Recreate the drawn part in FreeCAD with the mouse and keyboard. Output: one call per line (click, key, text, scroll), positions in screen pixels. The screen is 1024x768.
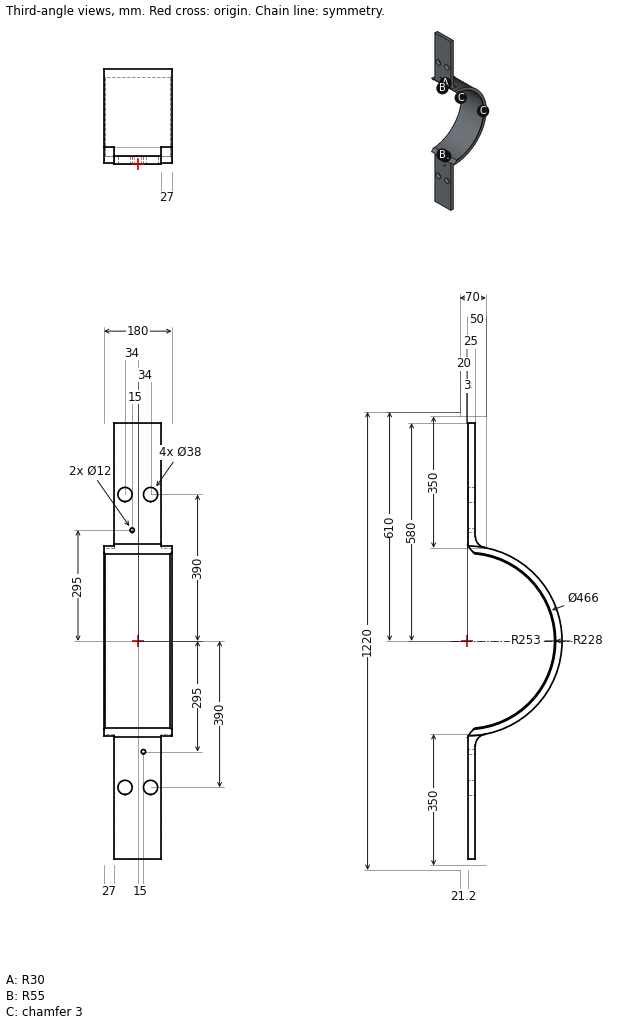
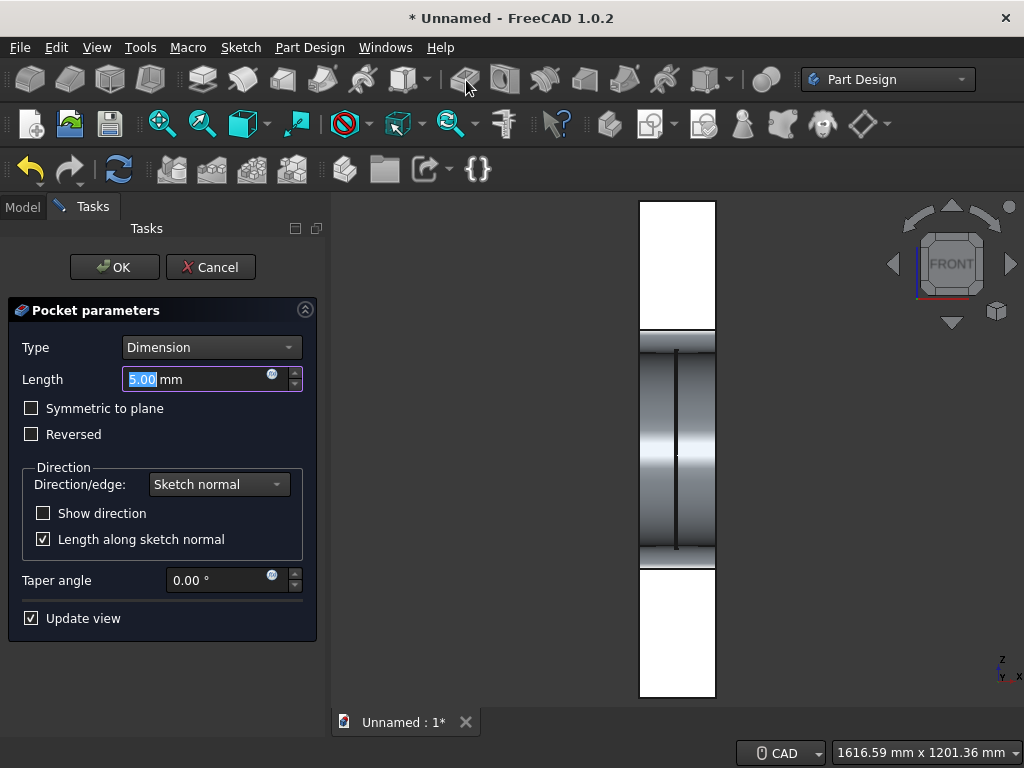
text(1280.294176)
key(Tab)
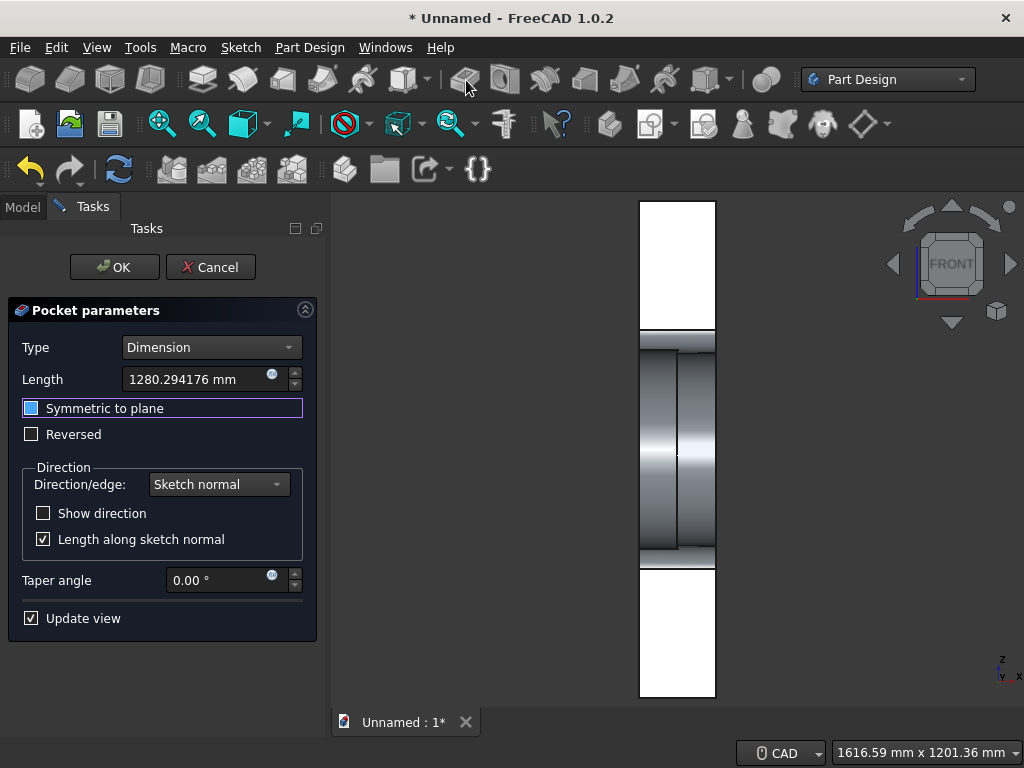
click(30, 408)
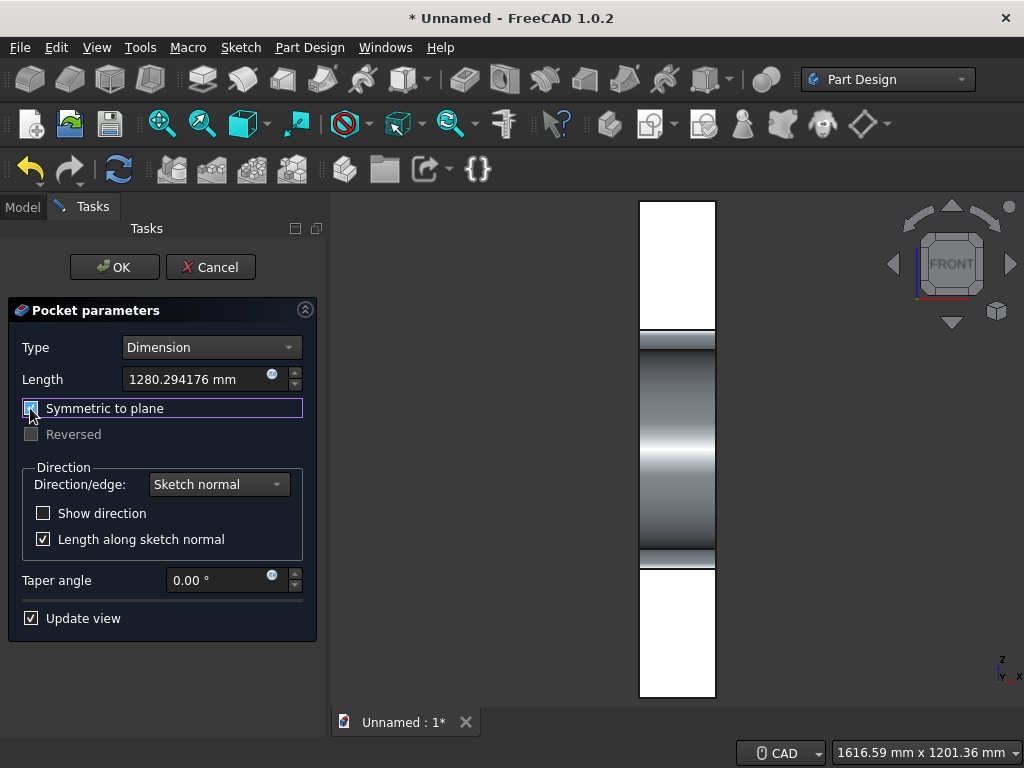
click(115, 267)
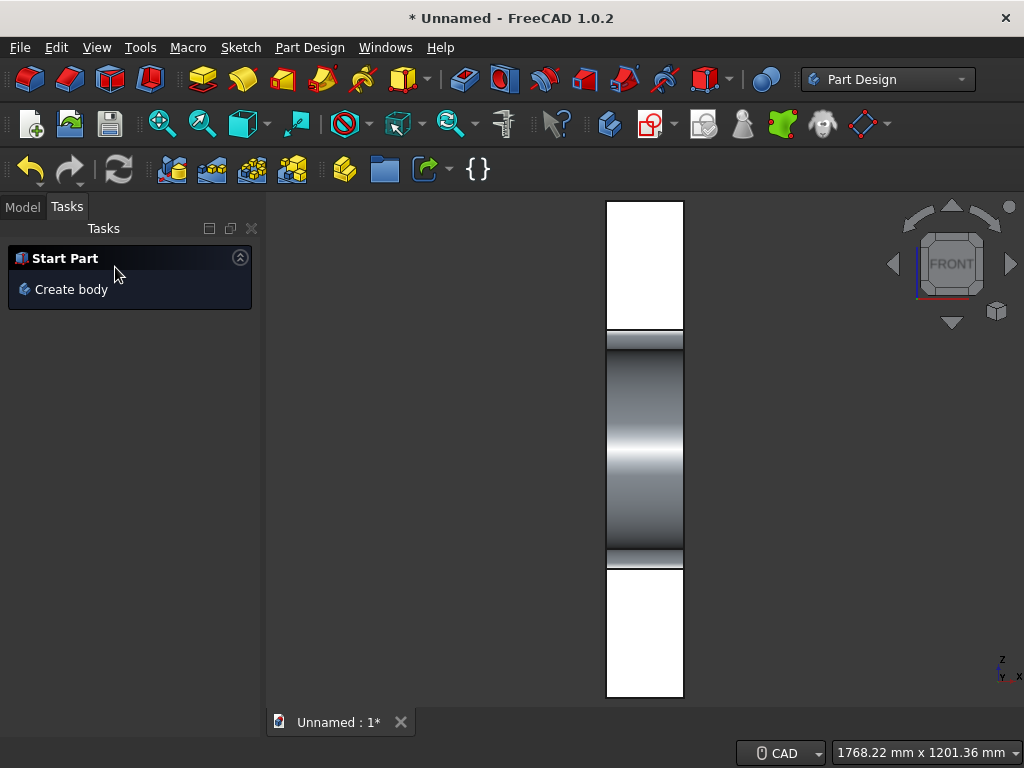
click(650, 124)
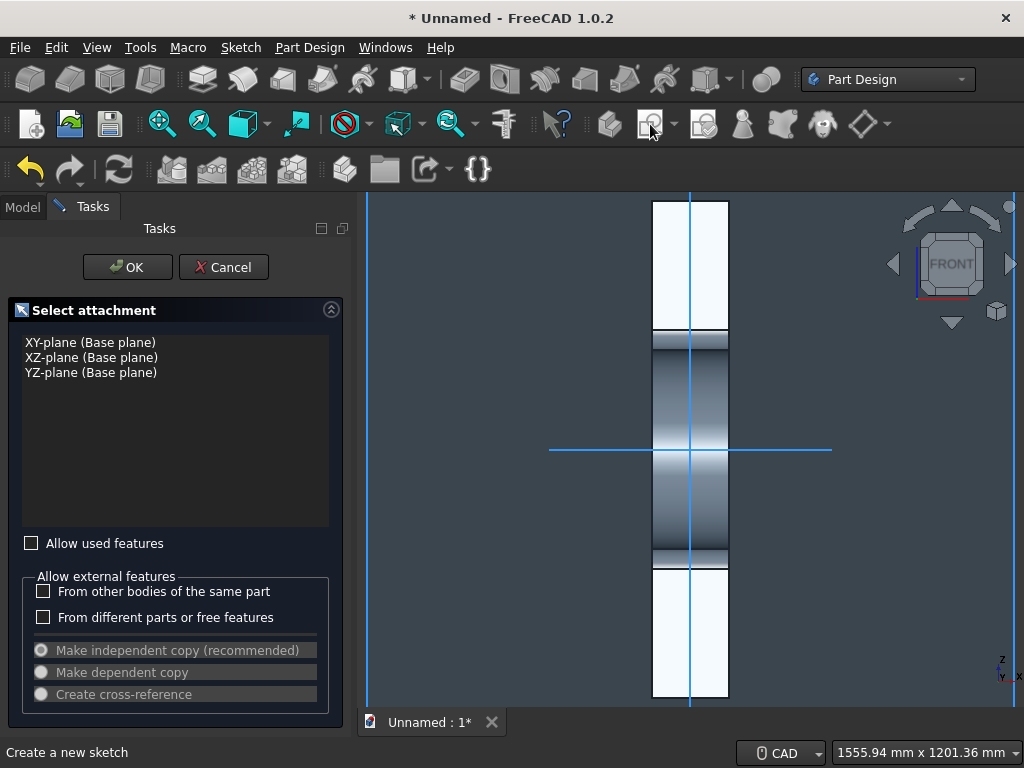
click(82, 372)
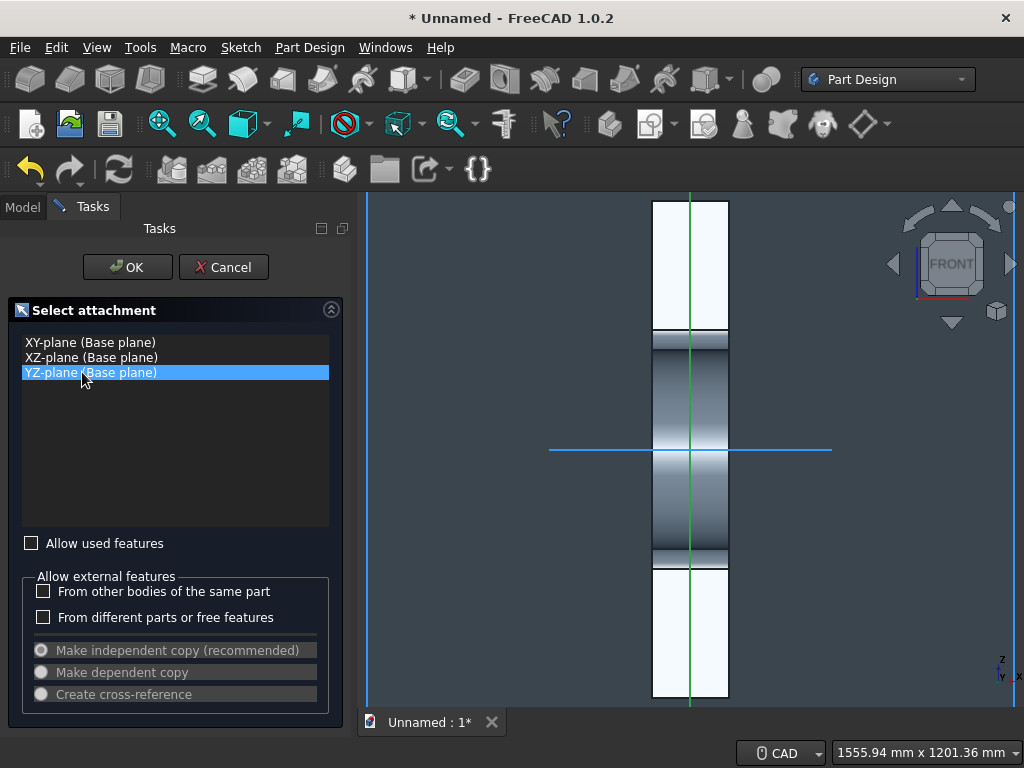
click(128, 267)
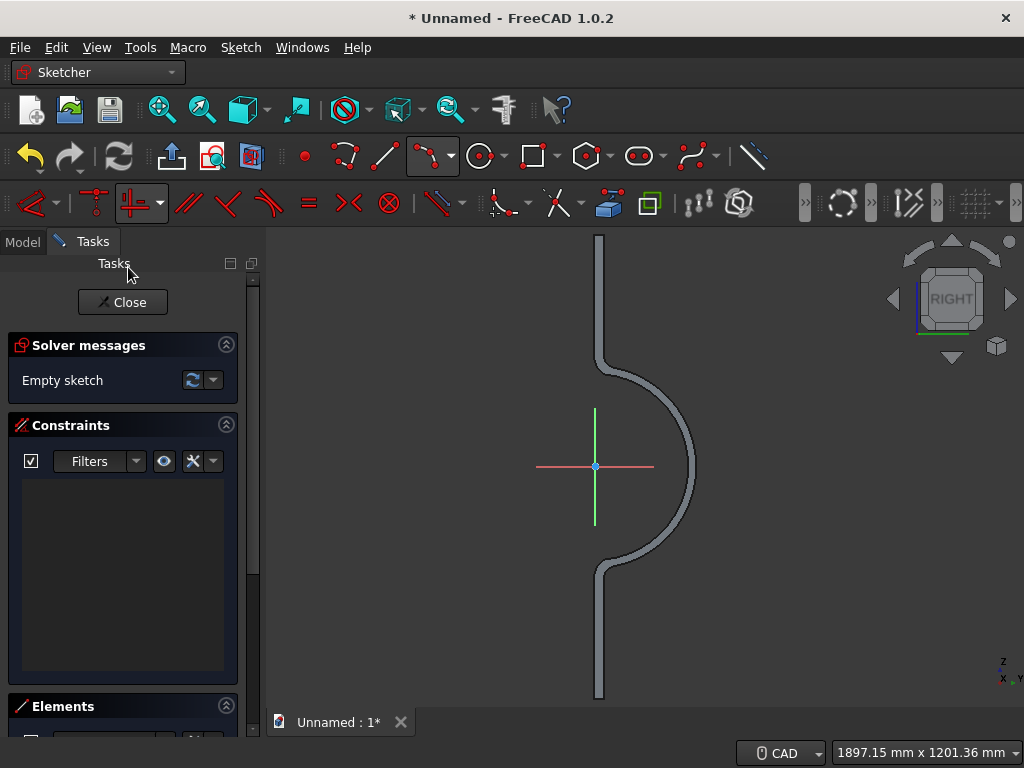
click(252, 156)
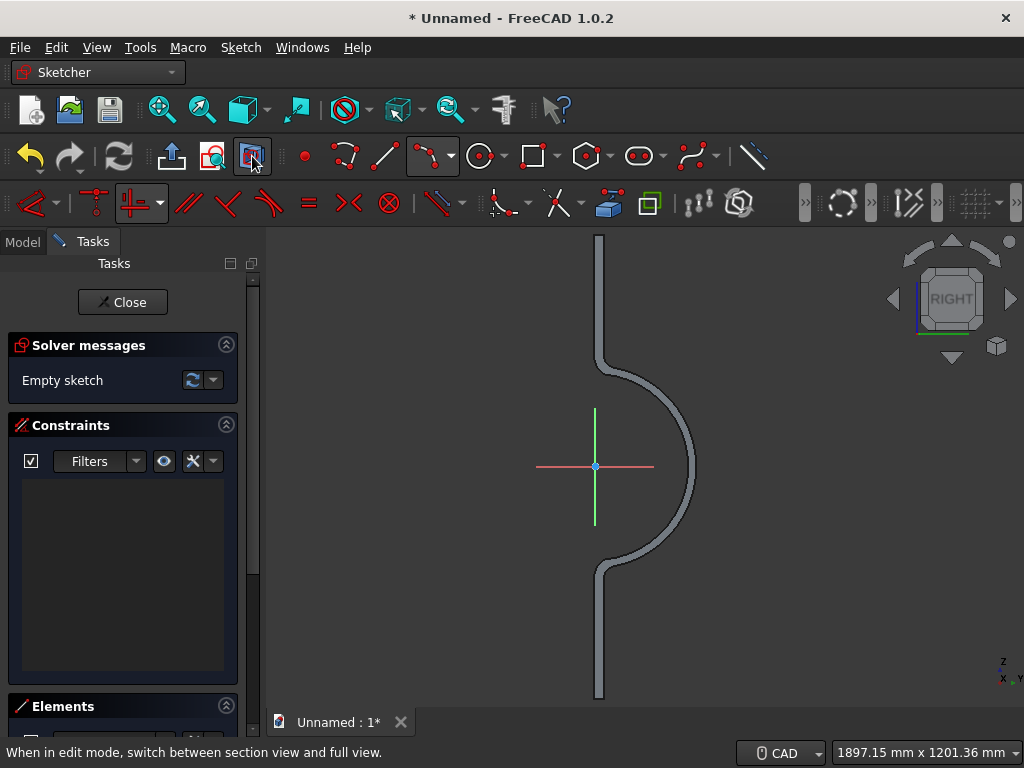
scroll(546, 467, down, 2)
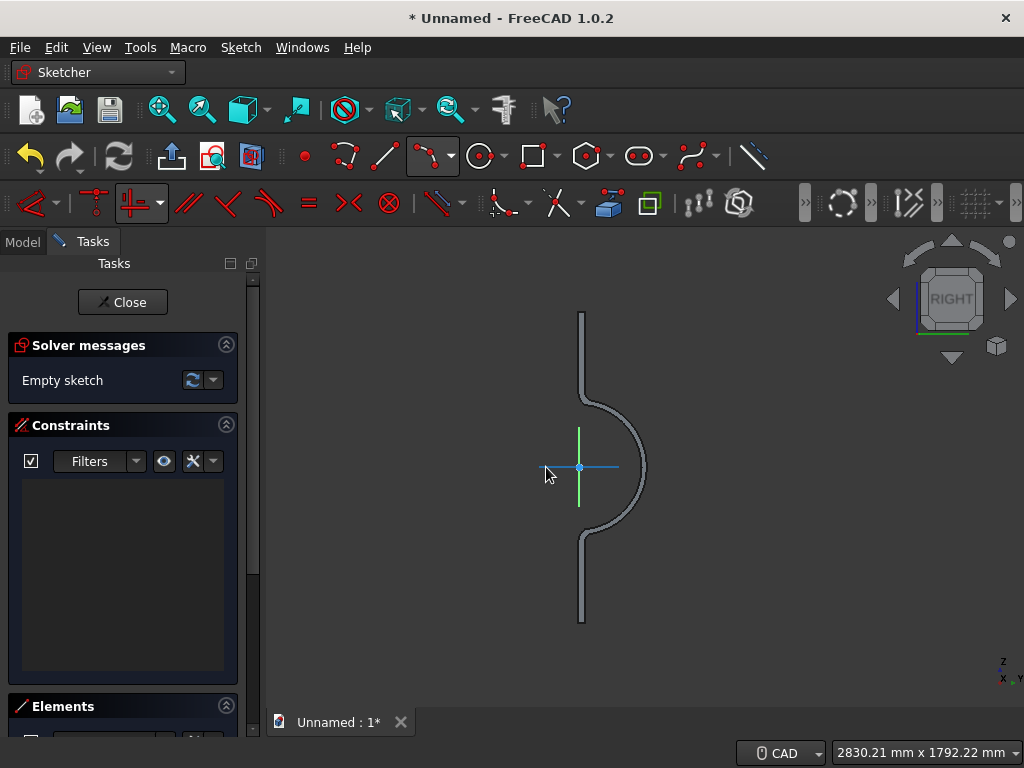
click(534, 156)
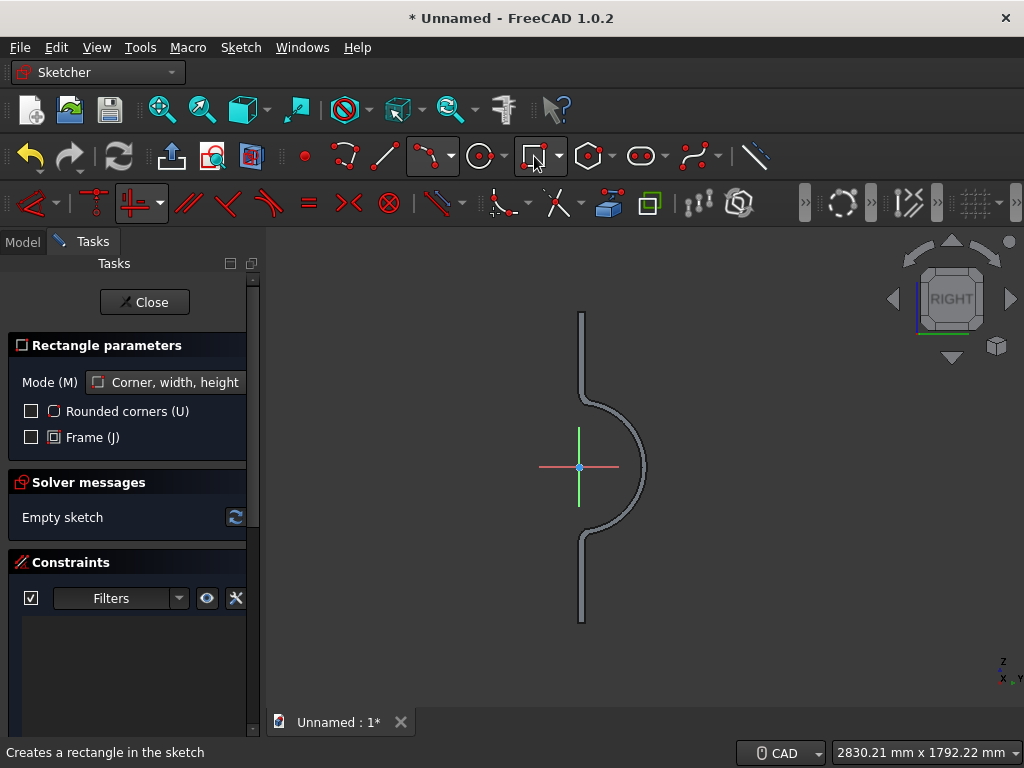
scroll(574, 304, up, 6)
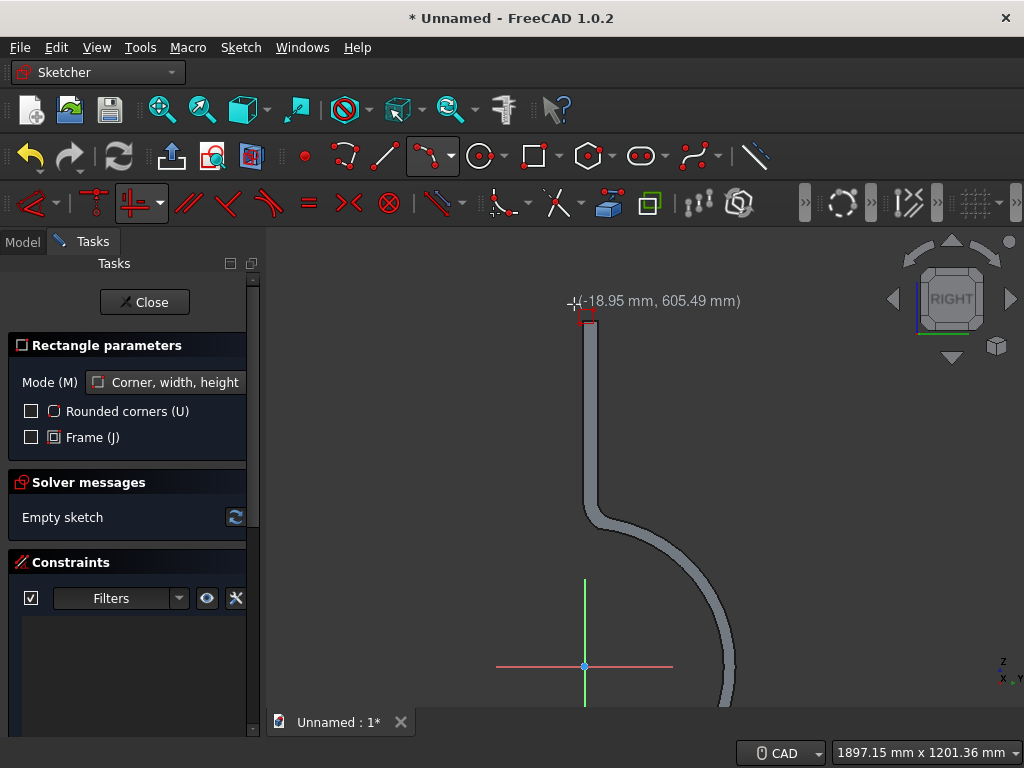
click(572, 303)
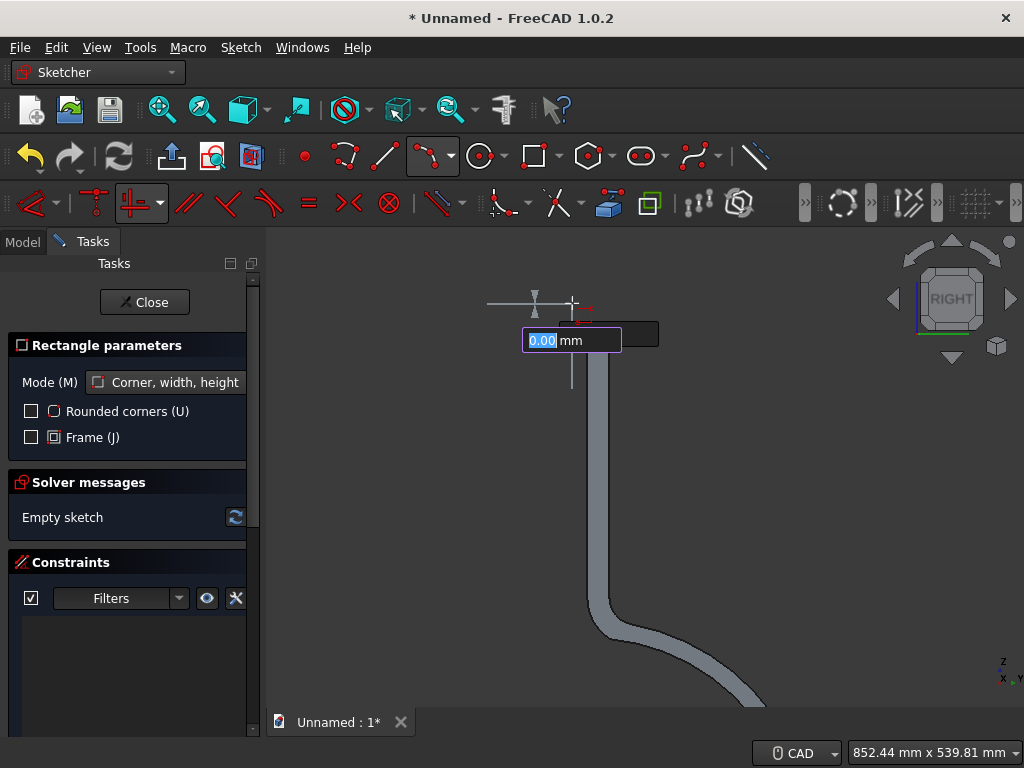
scroll(574, 304, down, 6)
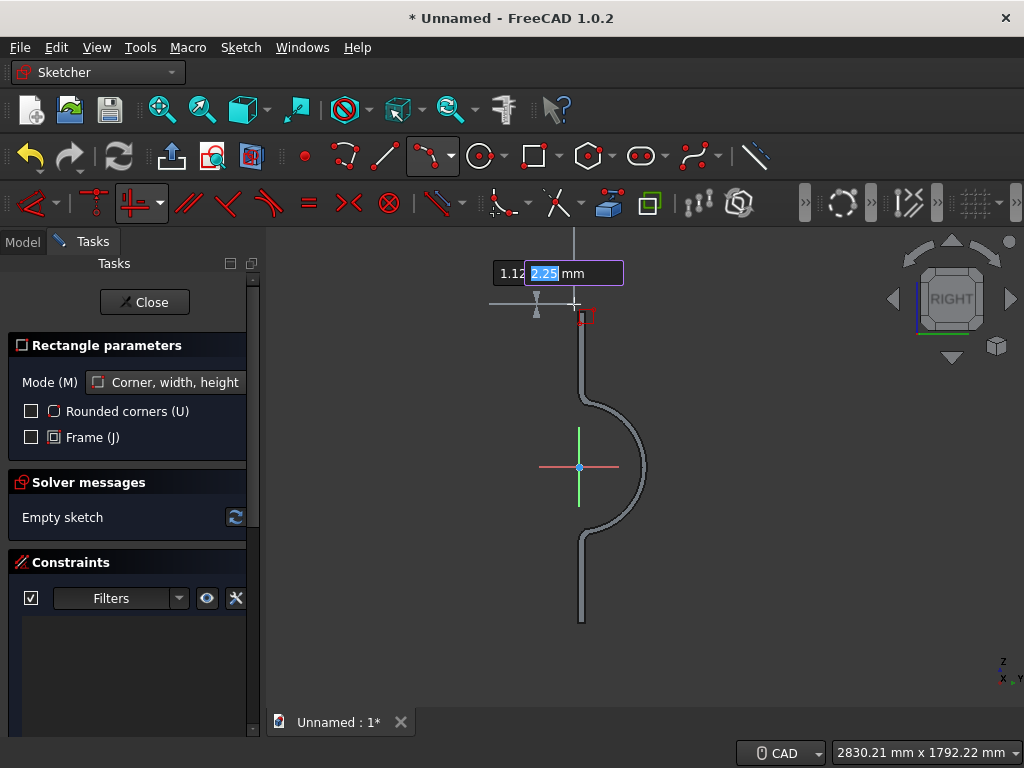
scroll(579, 631, up, 20)